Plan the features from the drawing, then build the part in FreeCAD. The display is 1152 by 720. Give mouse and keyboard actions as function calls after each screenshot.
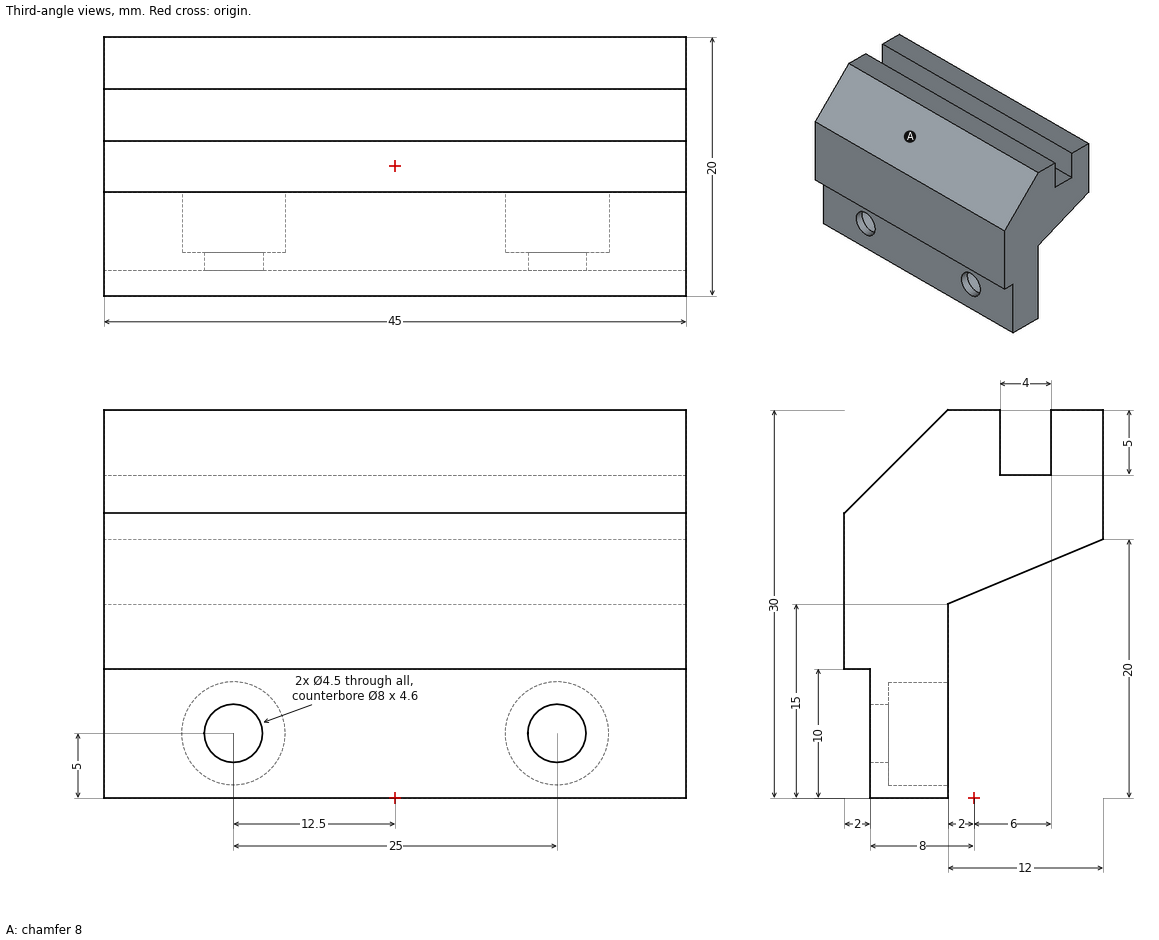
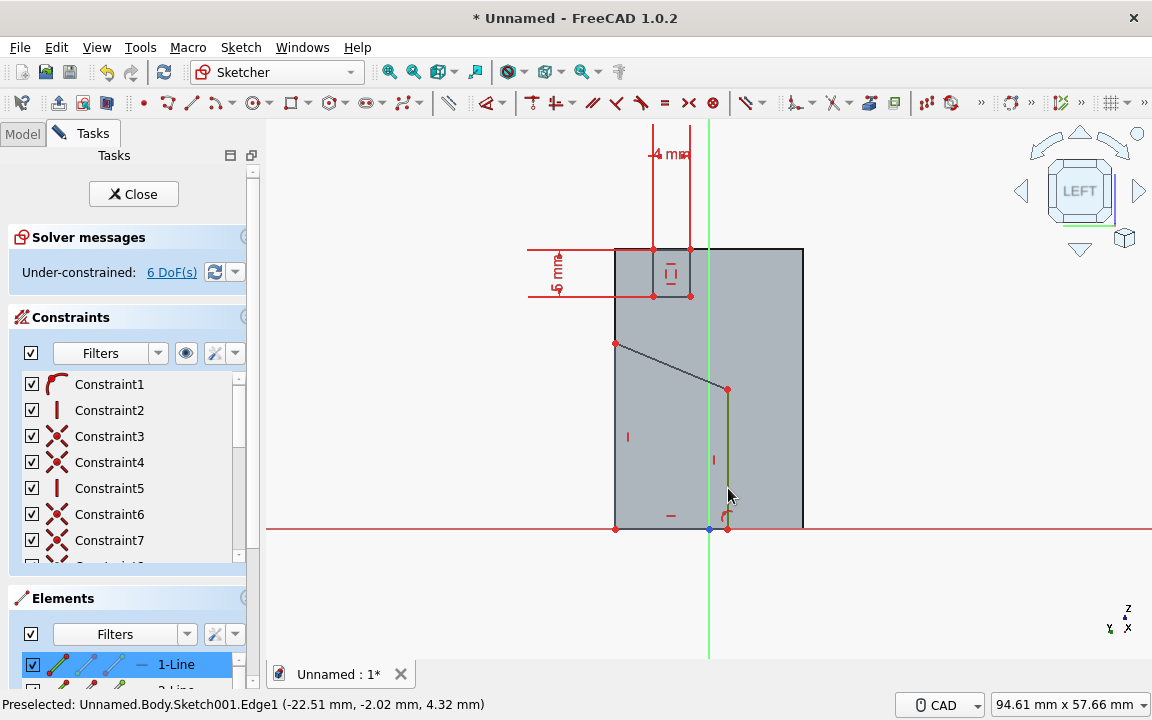
key(i)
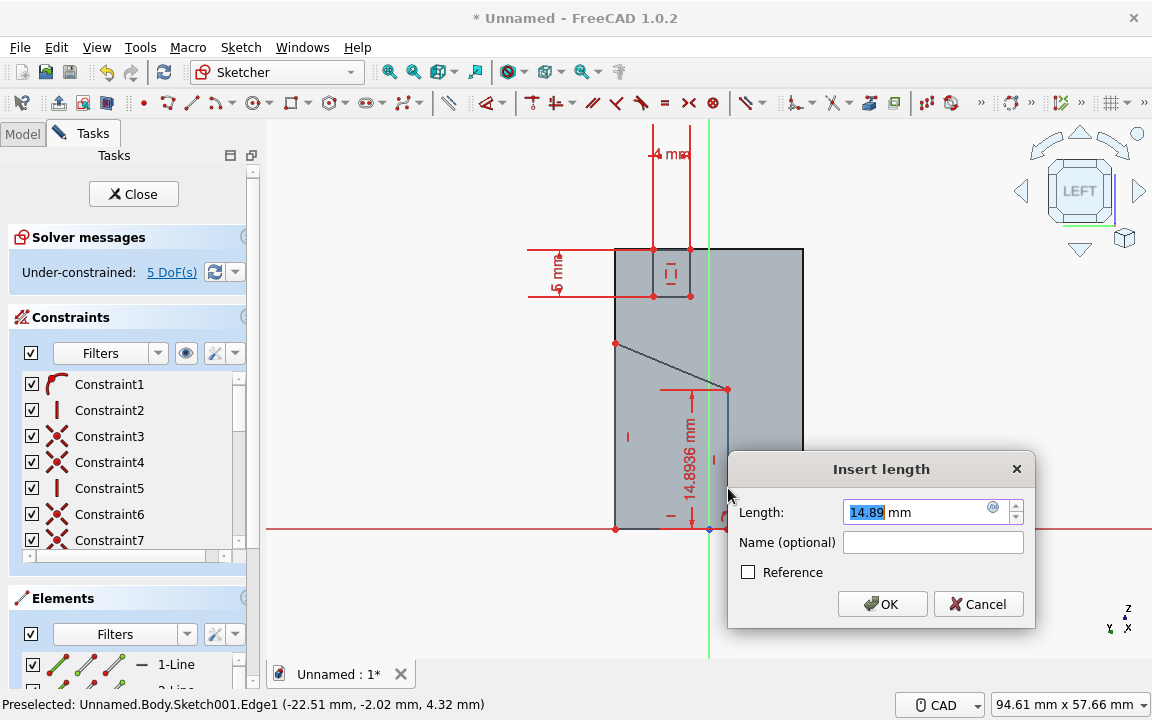
text(15)
key(Return)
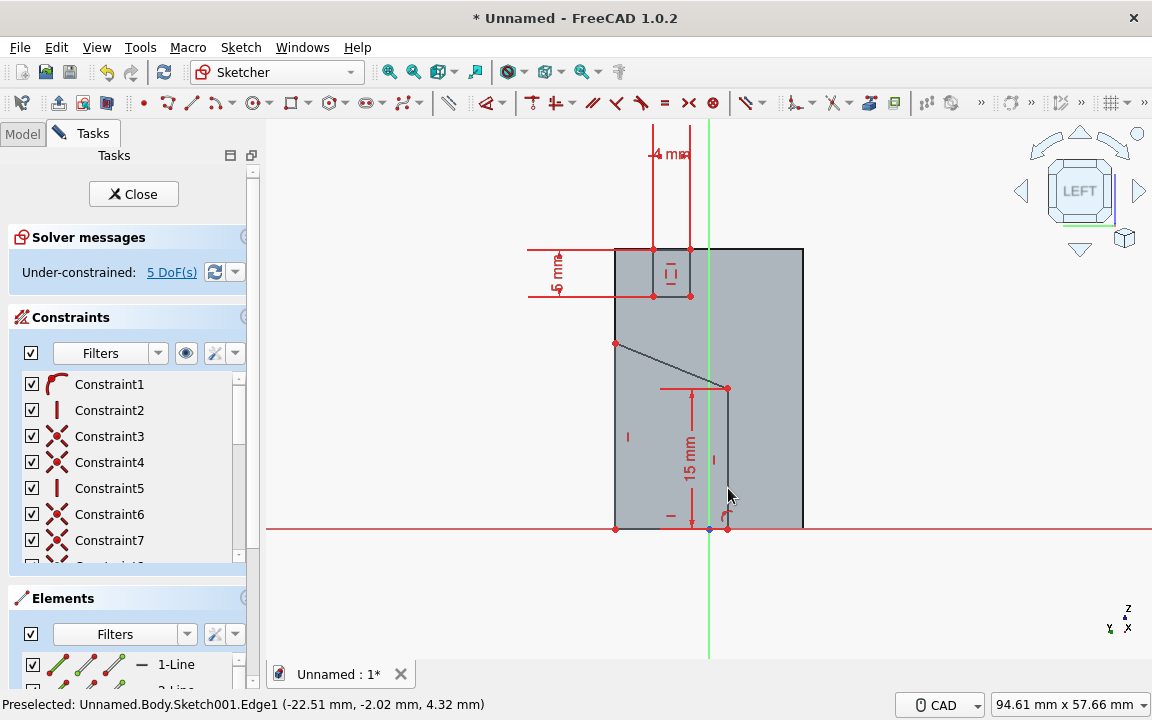
click(615, 399)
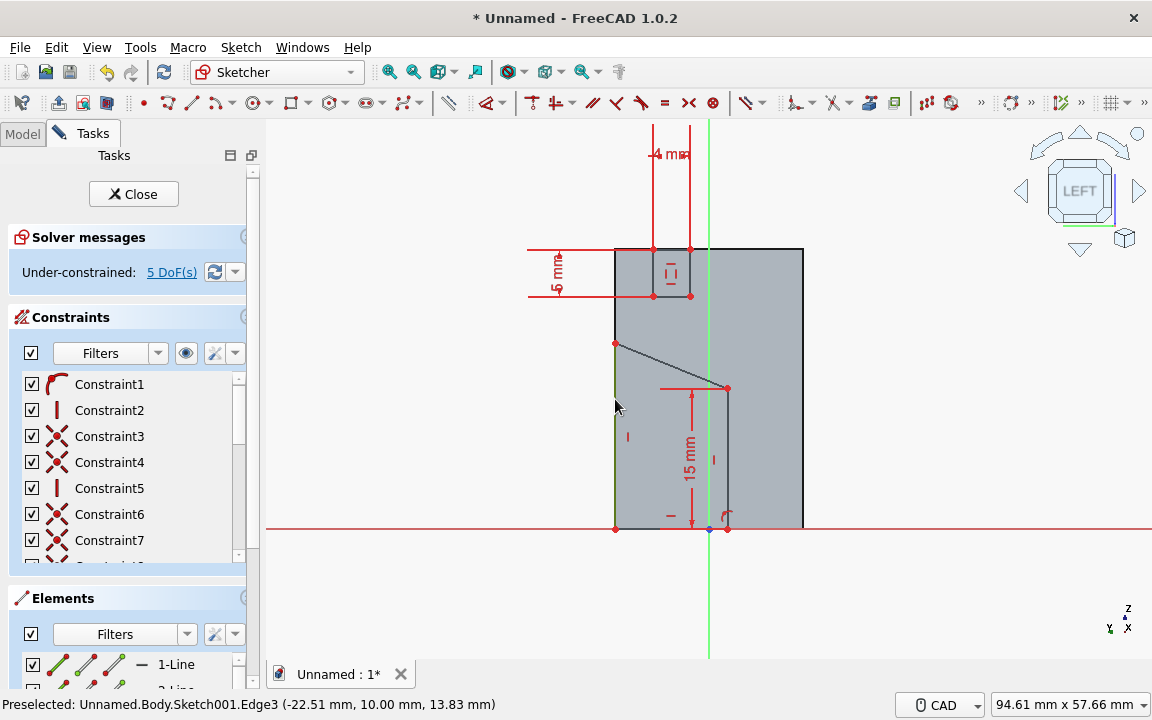
key(i)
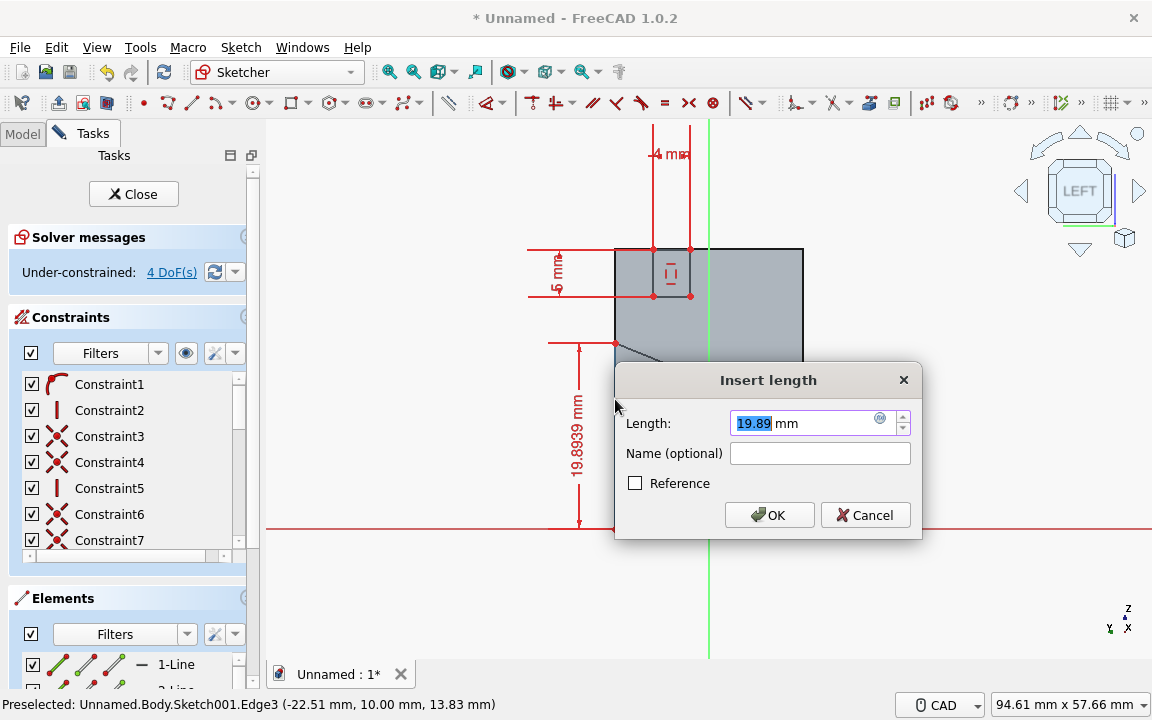
text(20)
key(Return)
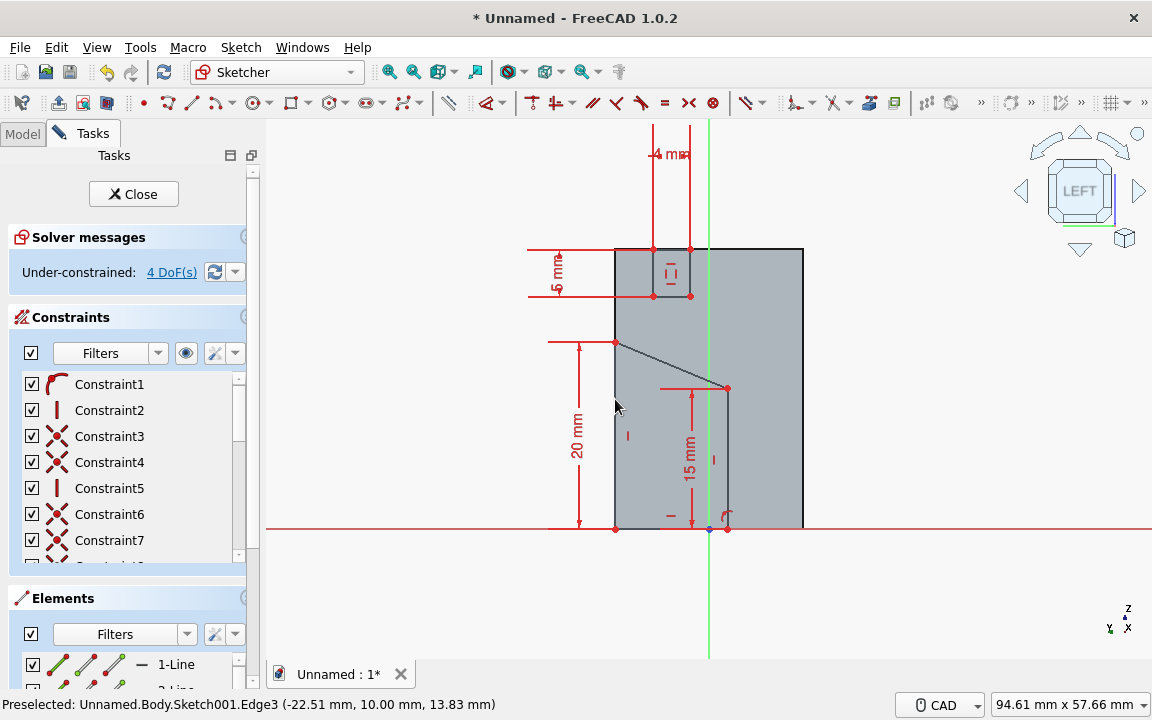
click(649, 529)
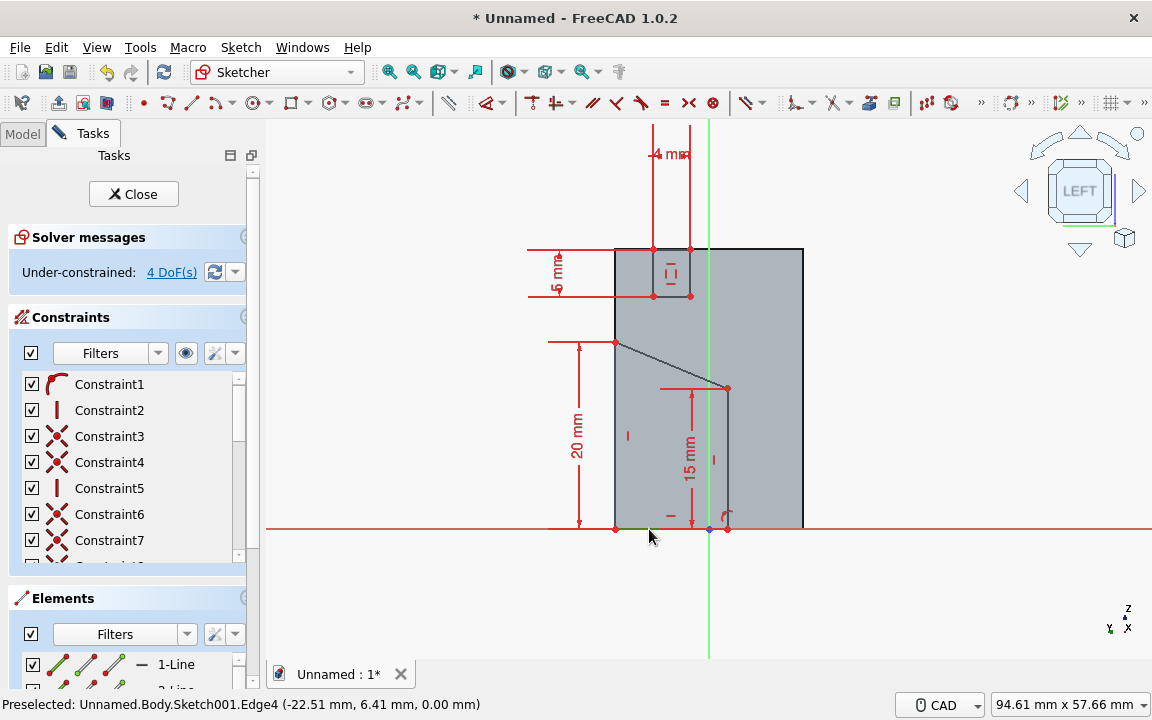
click(504, 104)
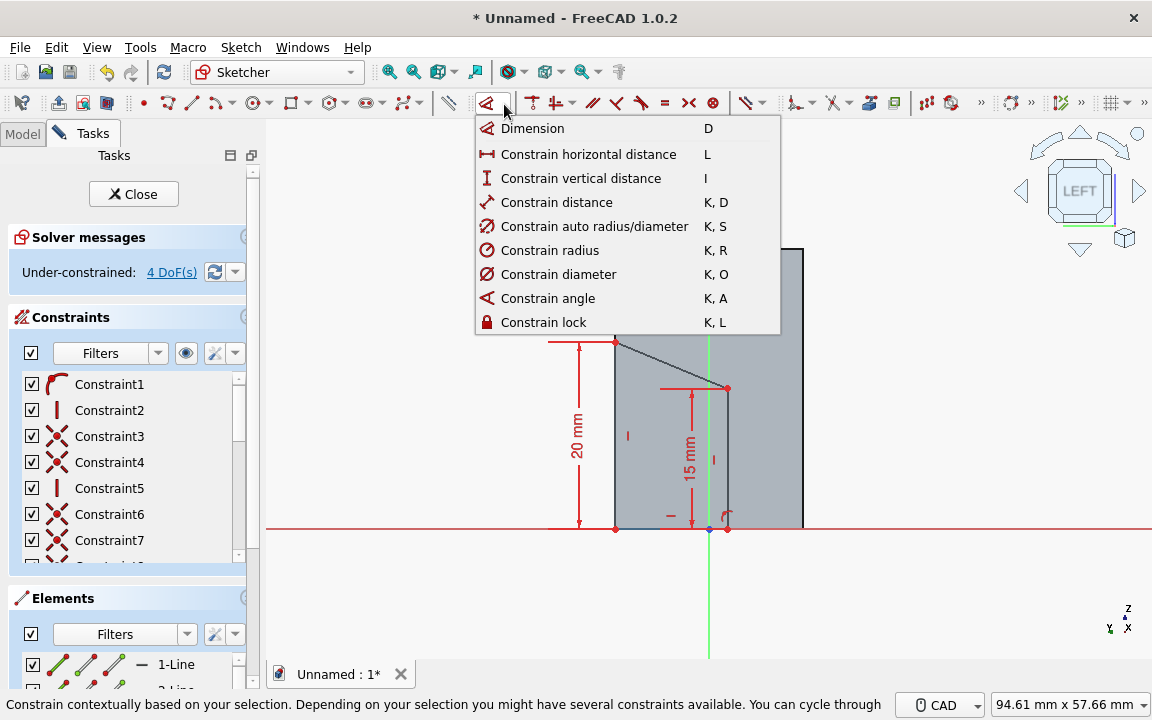
click(628, 154)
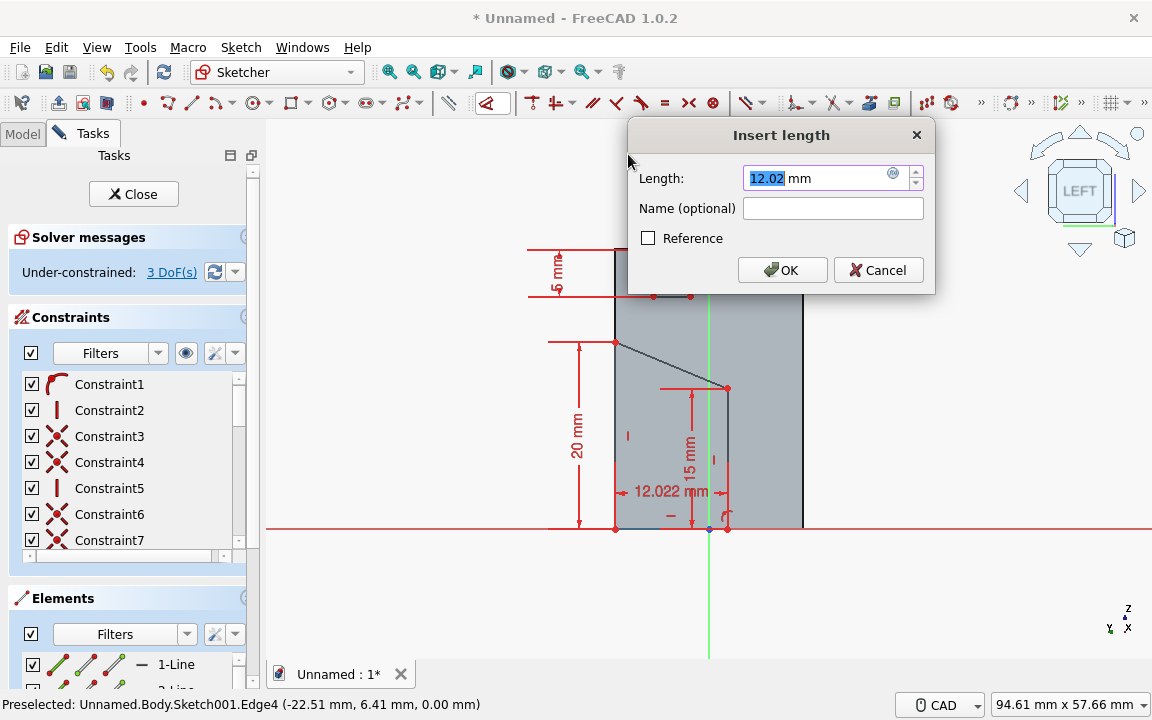
text(12)
key(Return)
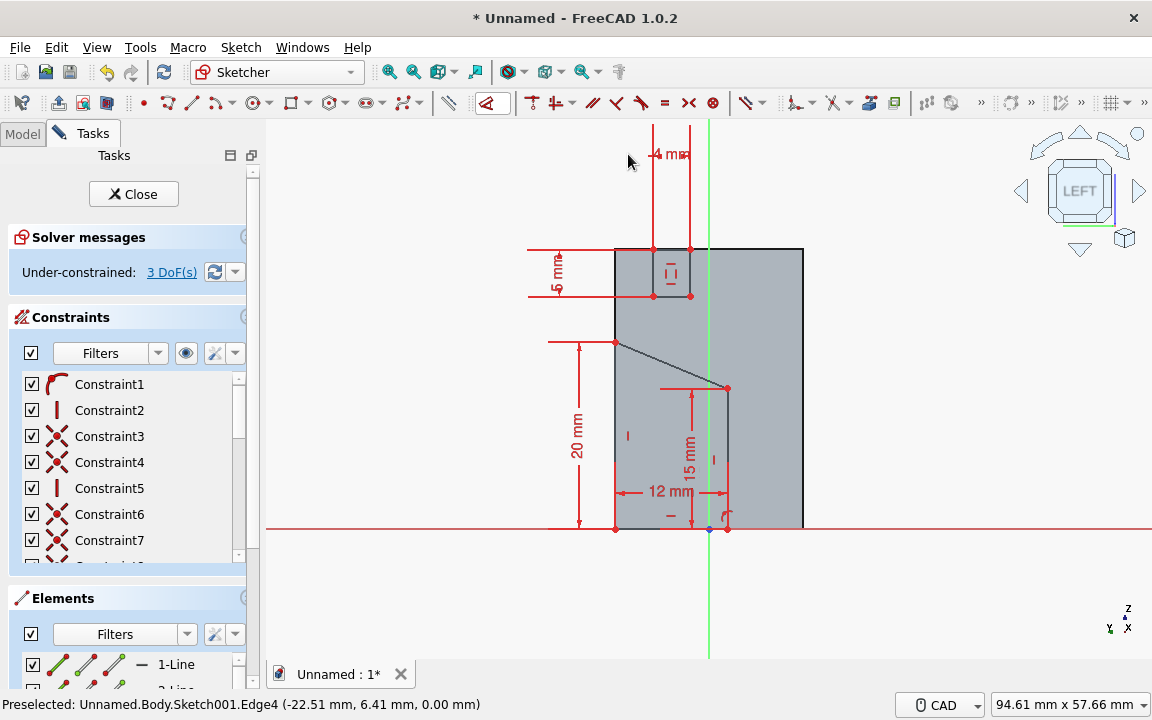
scroll(728, 529, up, 4)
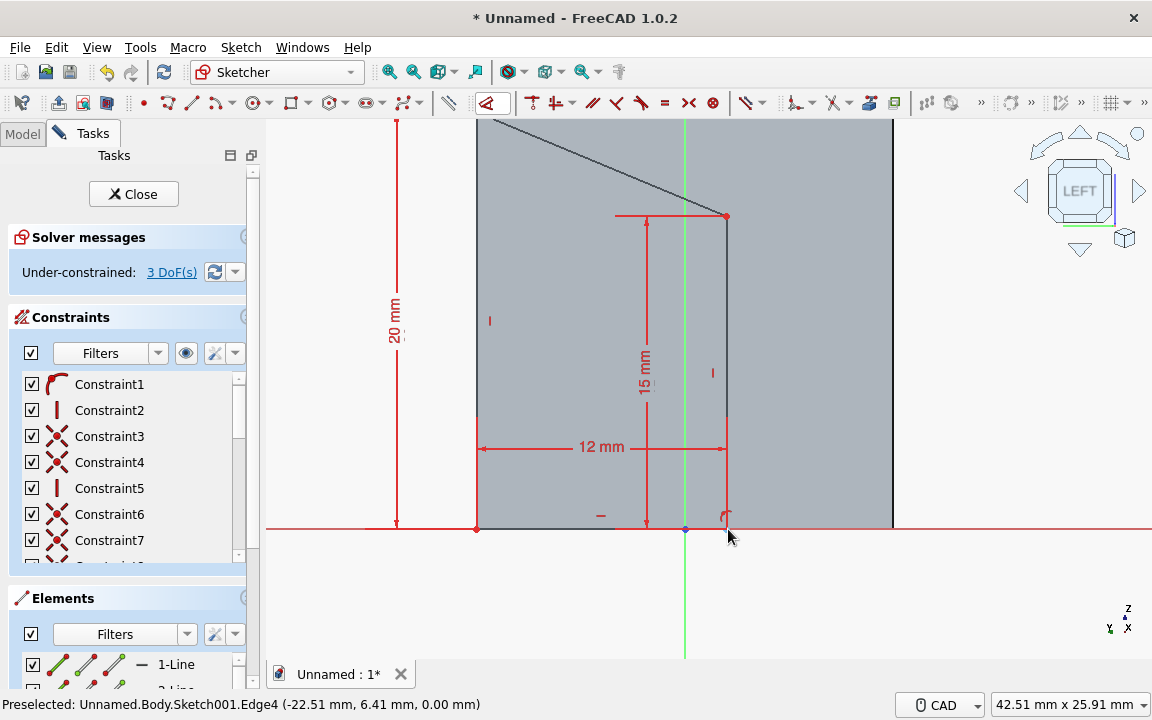
click(727, 529)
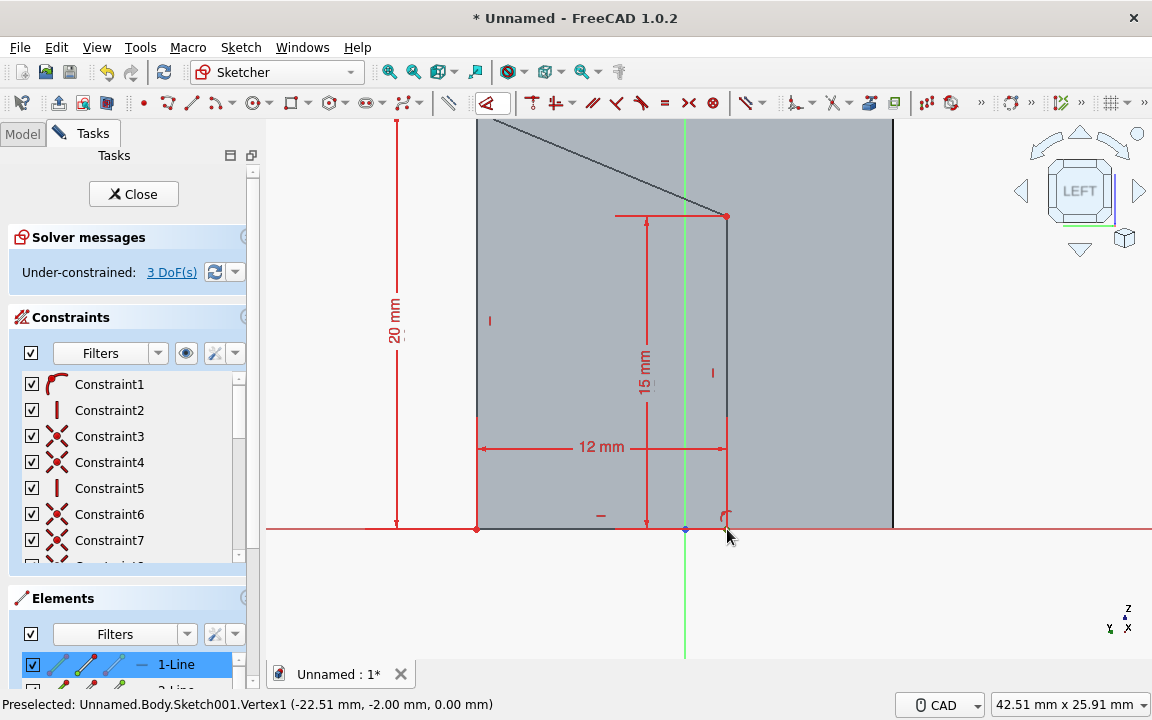
click(504, 104)